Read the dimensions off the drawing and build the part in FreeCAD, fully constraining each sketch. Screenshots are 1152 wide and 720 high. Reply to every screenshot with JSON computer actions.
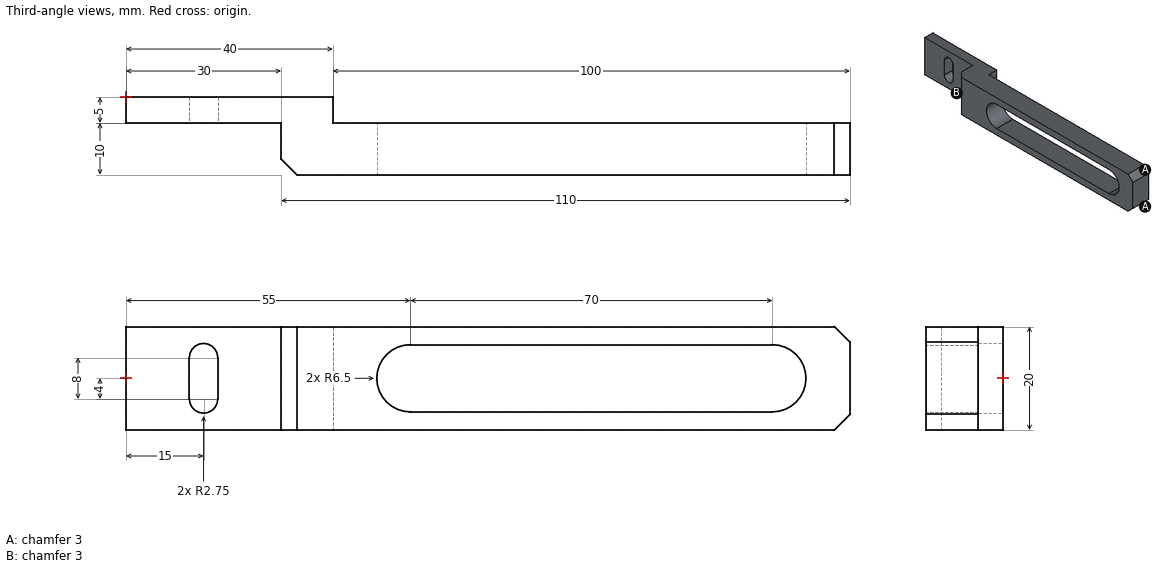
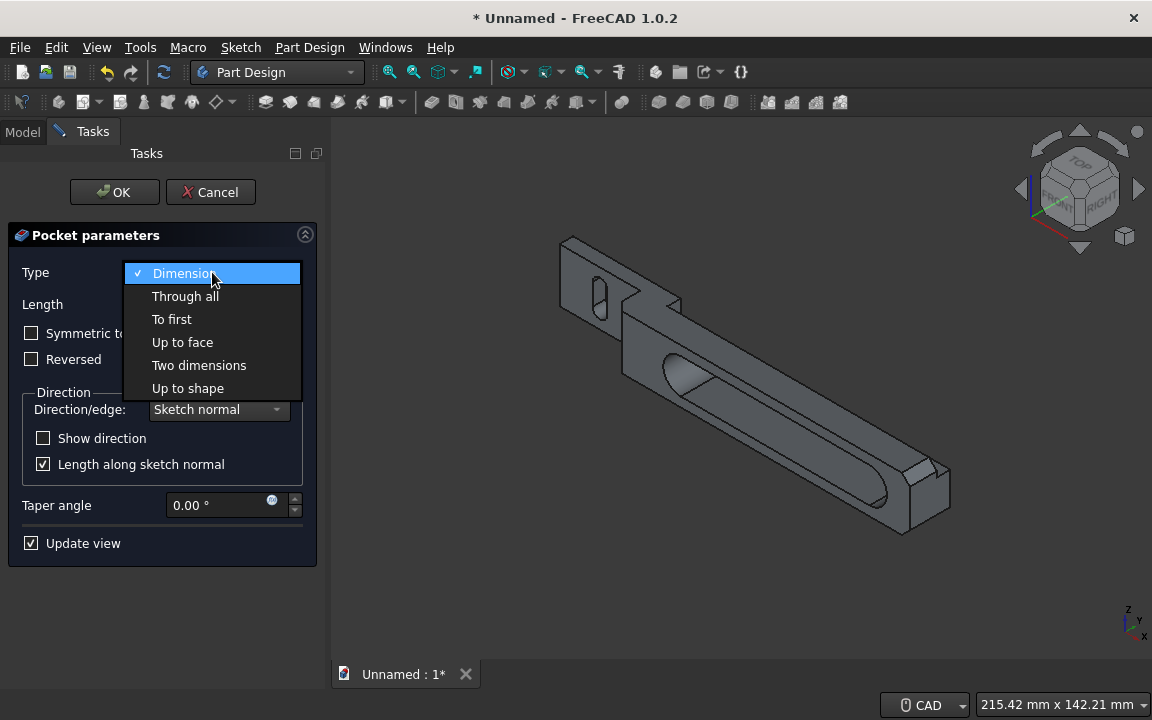
{"action": "left_click", "coordinate": [212, 296]}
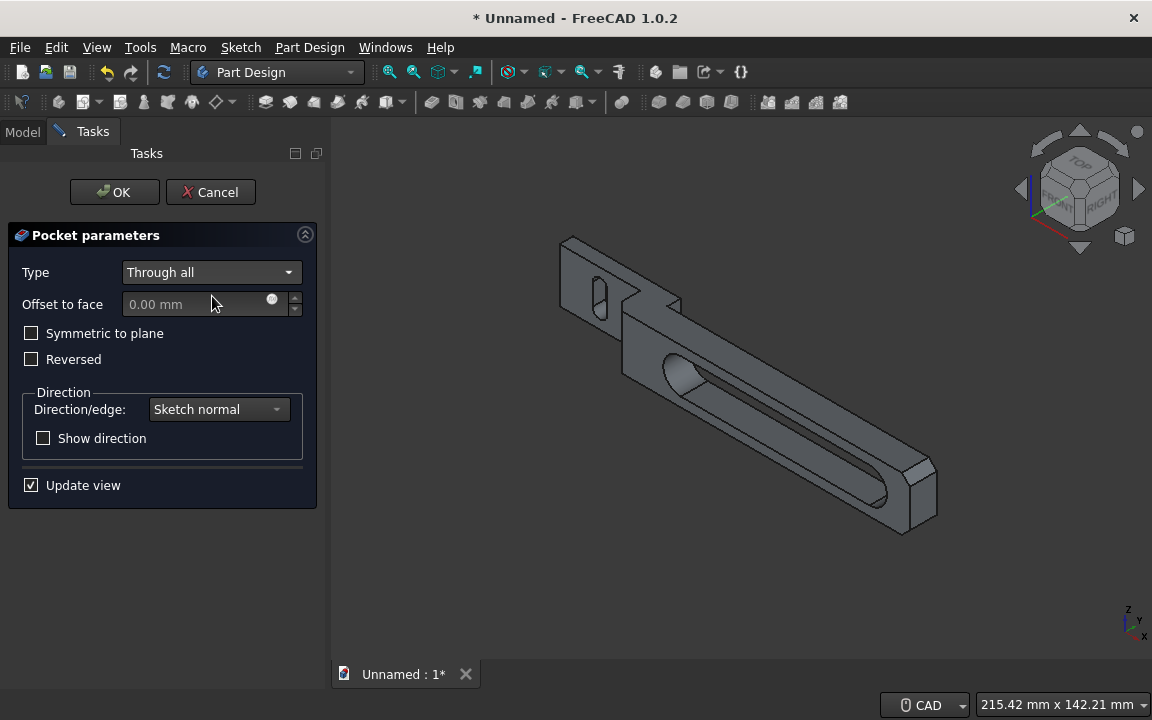
{"action": "left_click", "coordinate": [115, 192]}